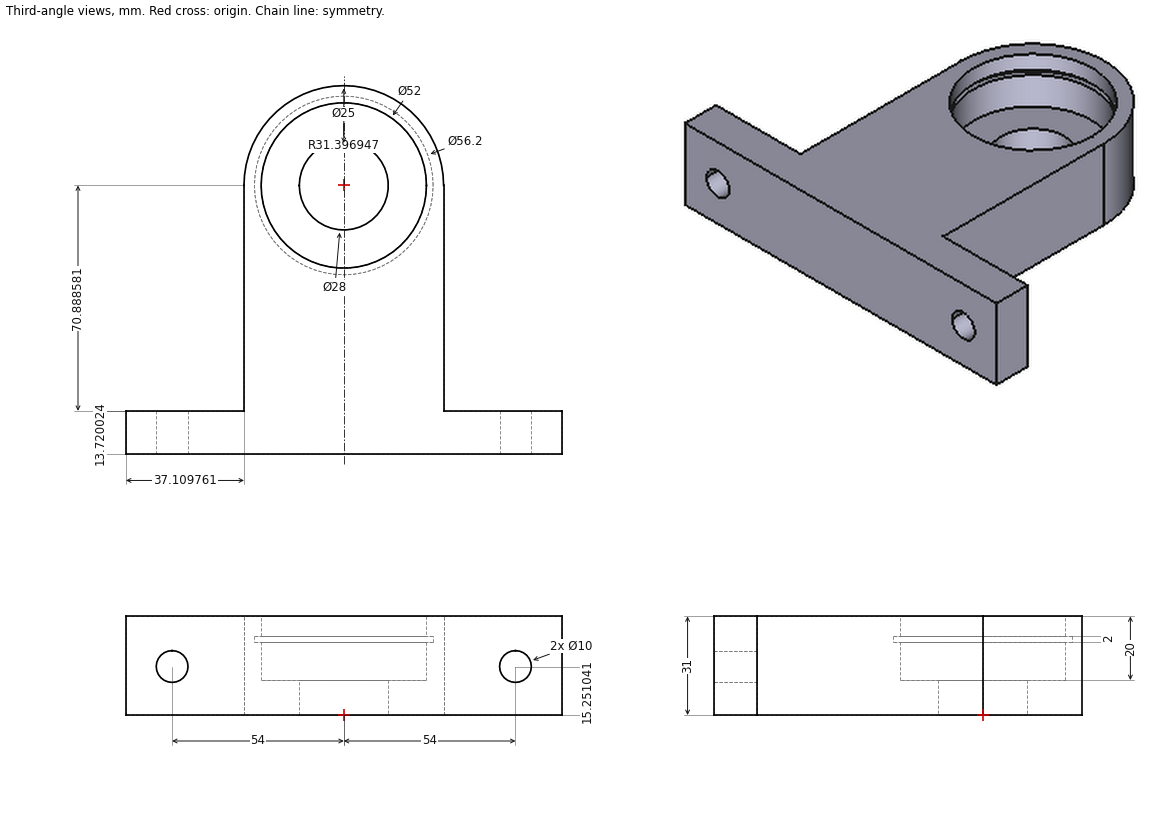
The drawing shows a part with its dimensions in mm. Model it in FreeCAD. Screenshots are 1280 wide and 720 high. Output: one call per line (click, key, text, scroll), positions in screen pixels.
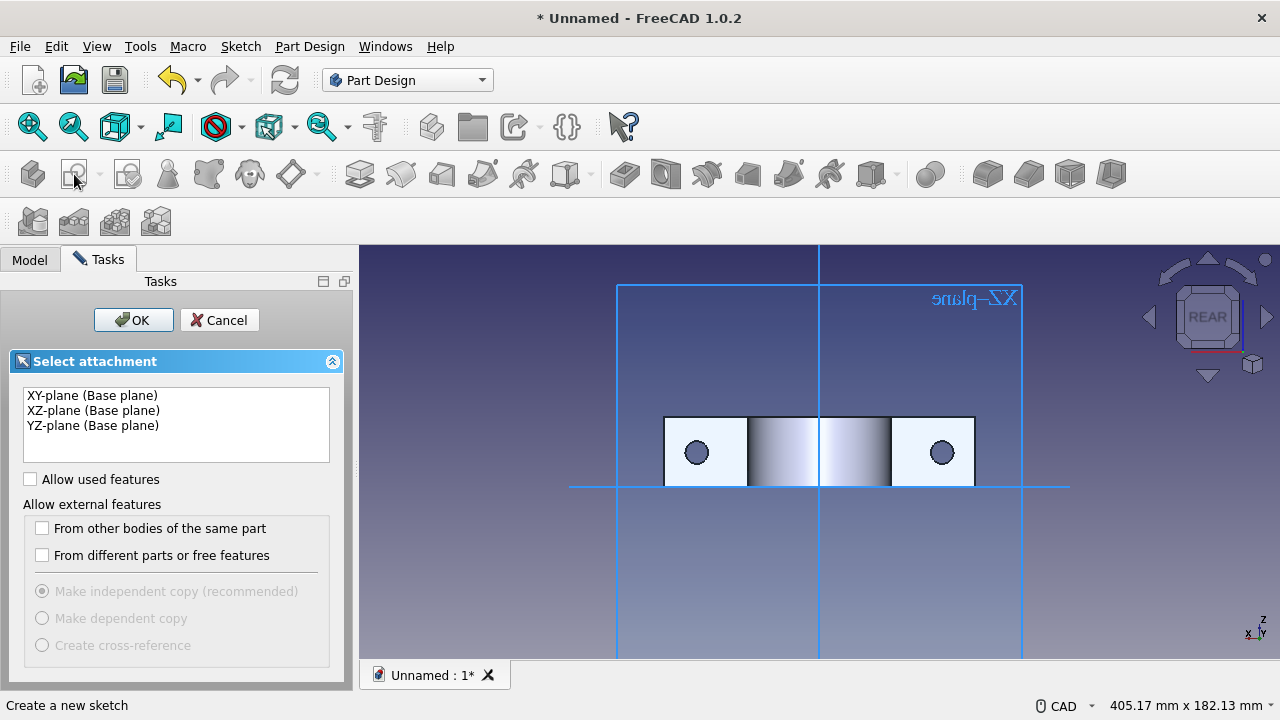
click(84, 396)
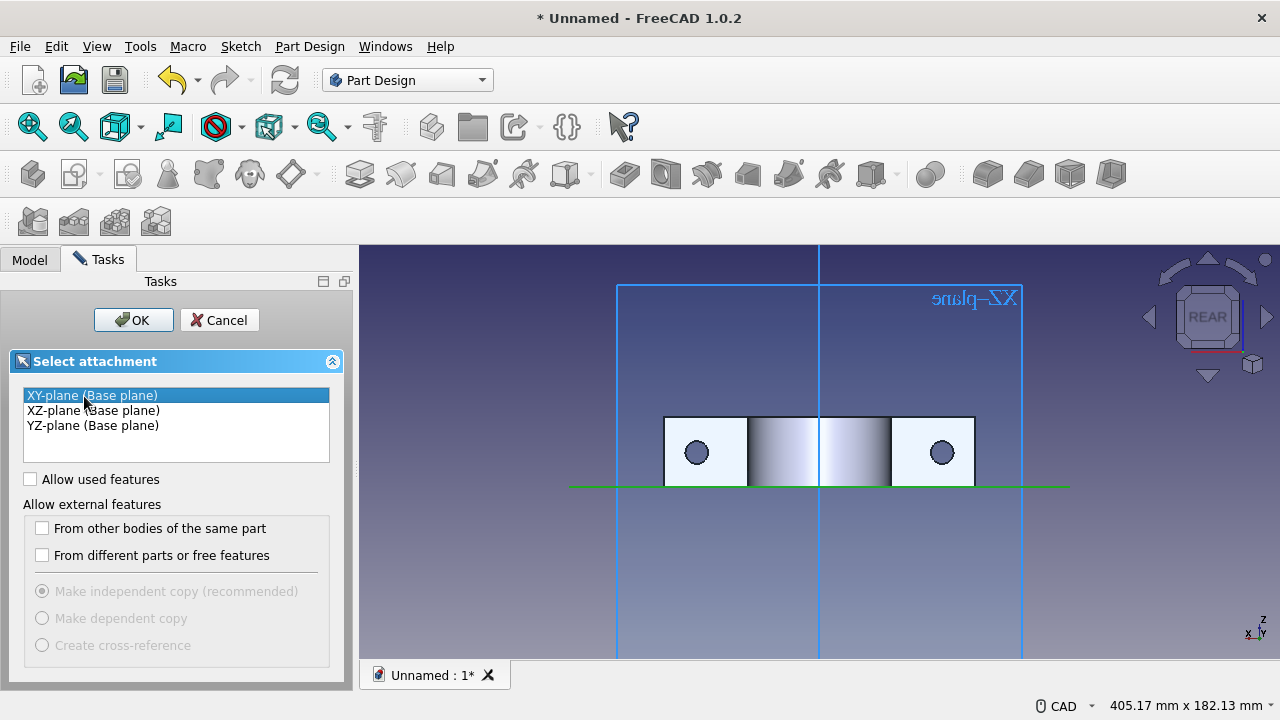
click(134, 320)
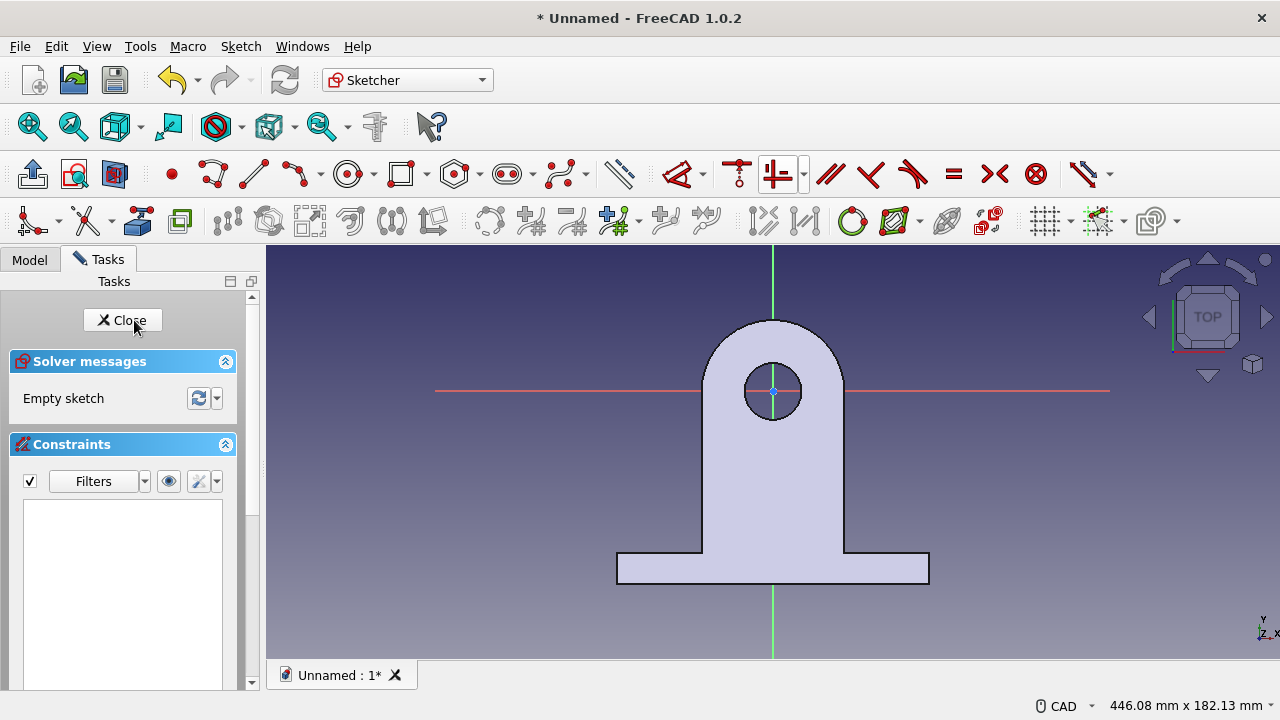
click(115, 174)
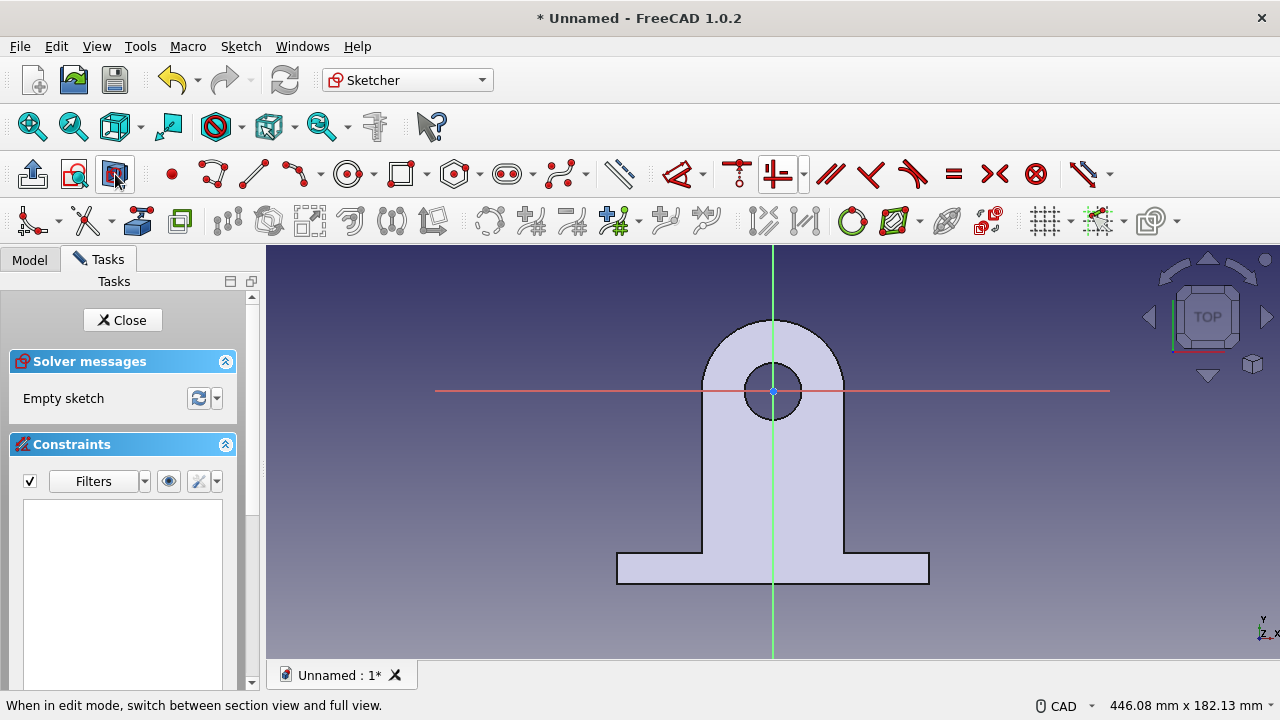
scroll(795, 372, up, 7)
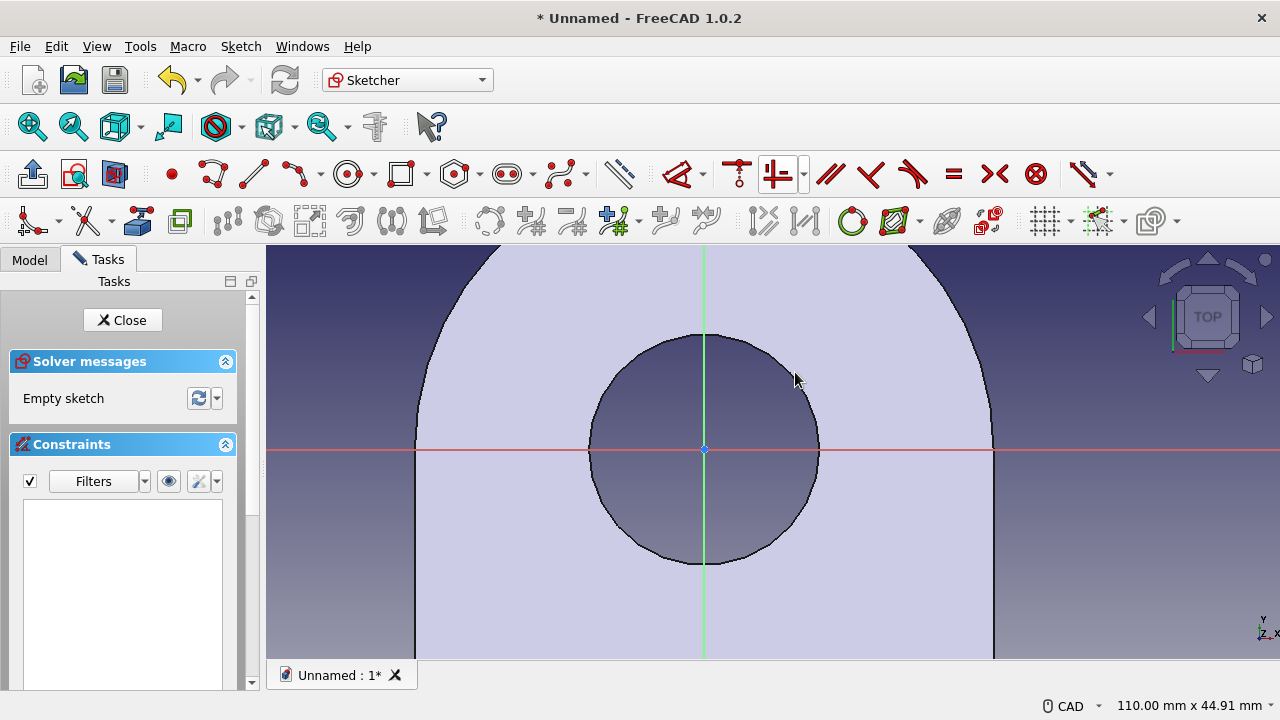
click(348, 174)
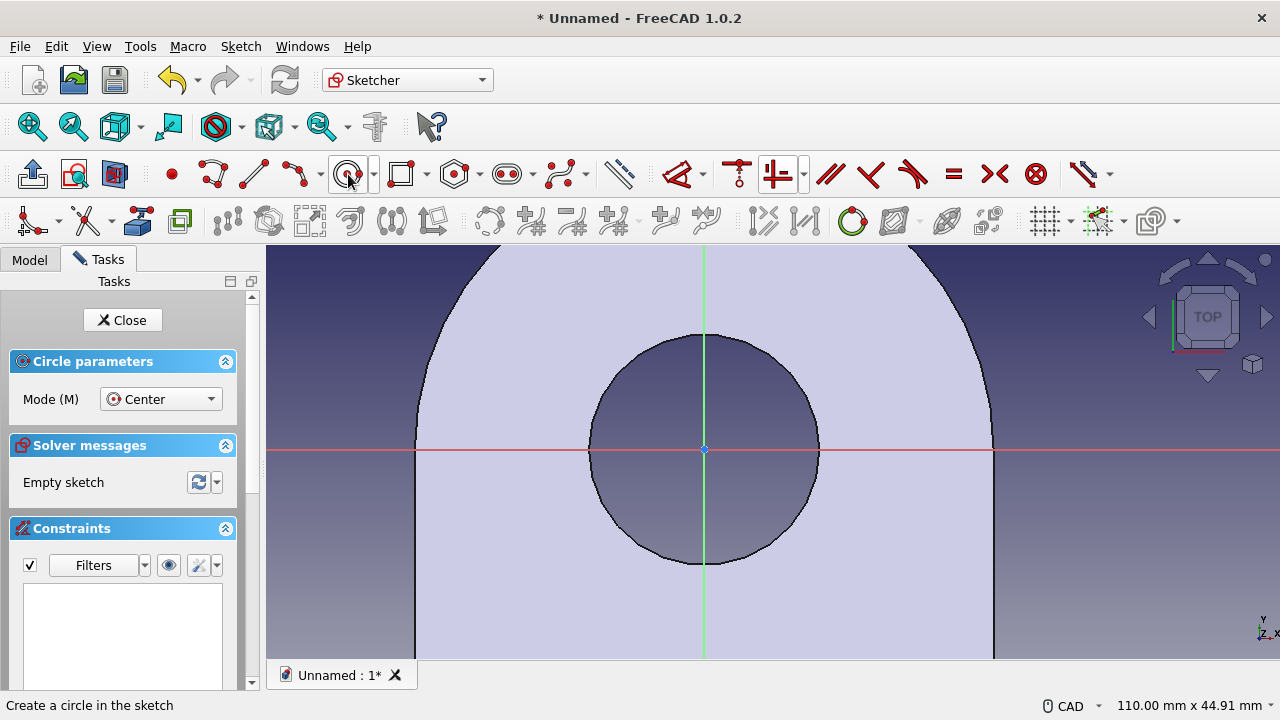
click(704, 450)
click(795, 359)
key(Escape)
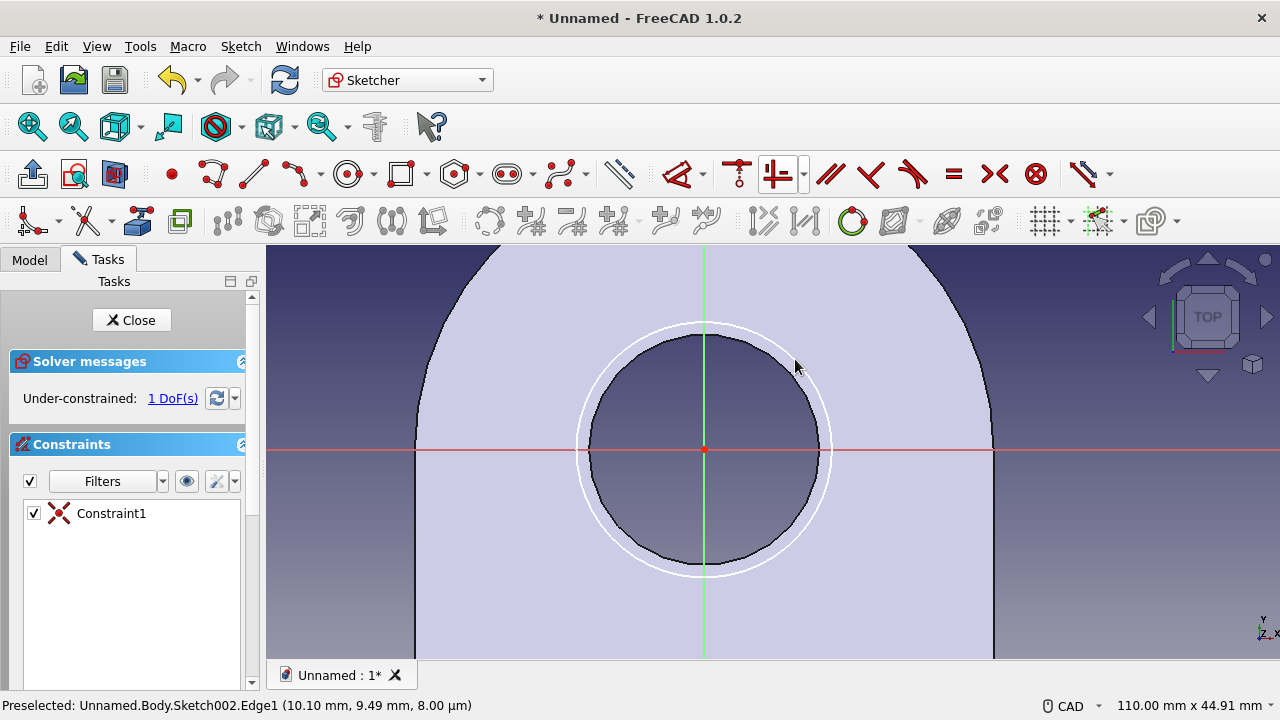
key(d)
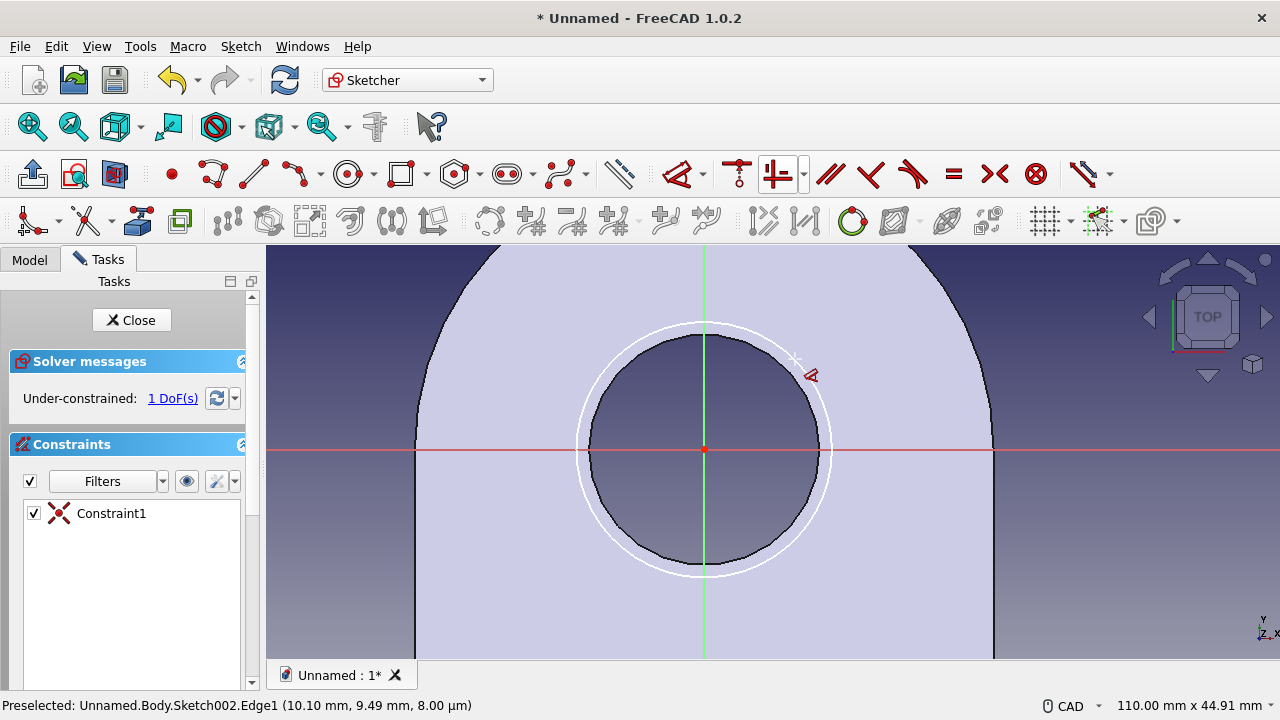
click(794, 359)
click(817, 336)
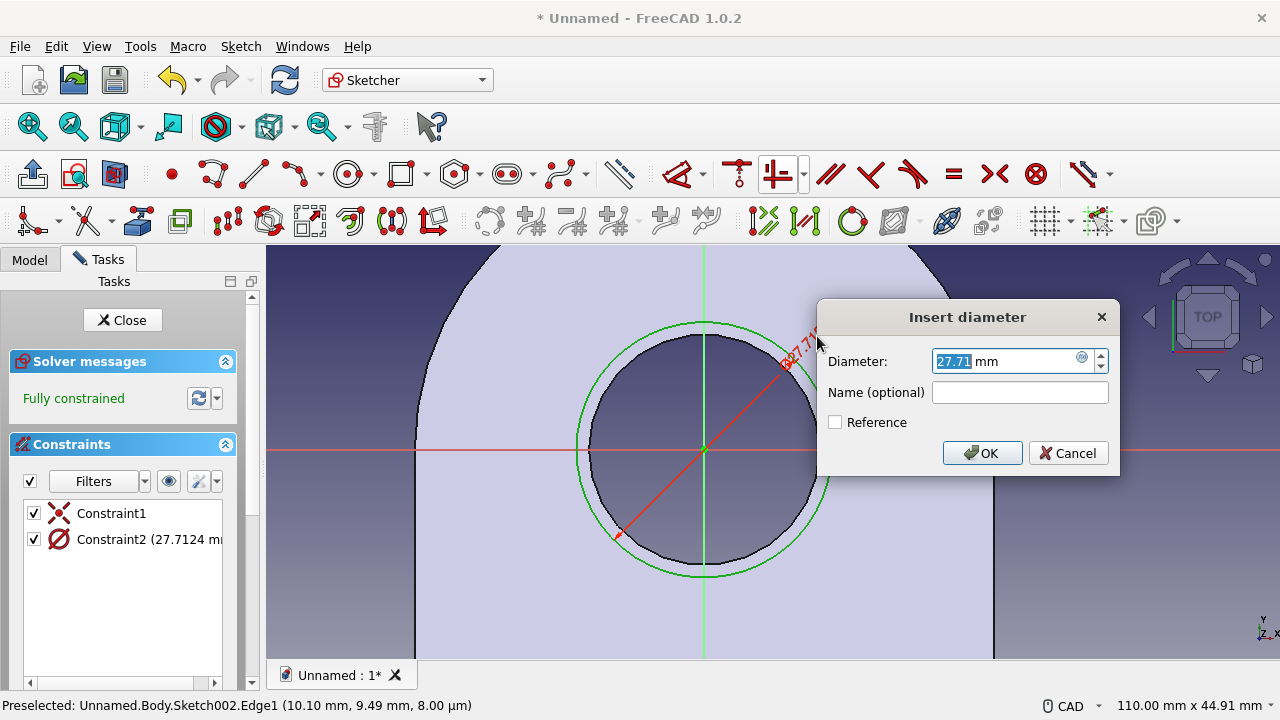
text(28)
key(Return)
key(Escape)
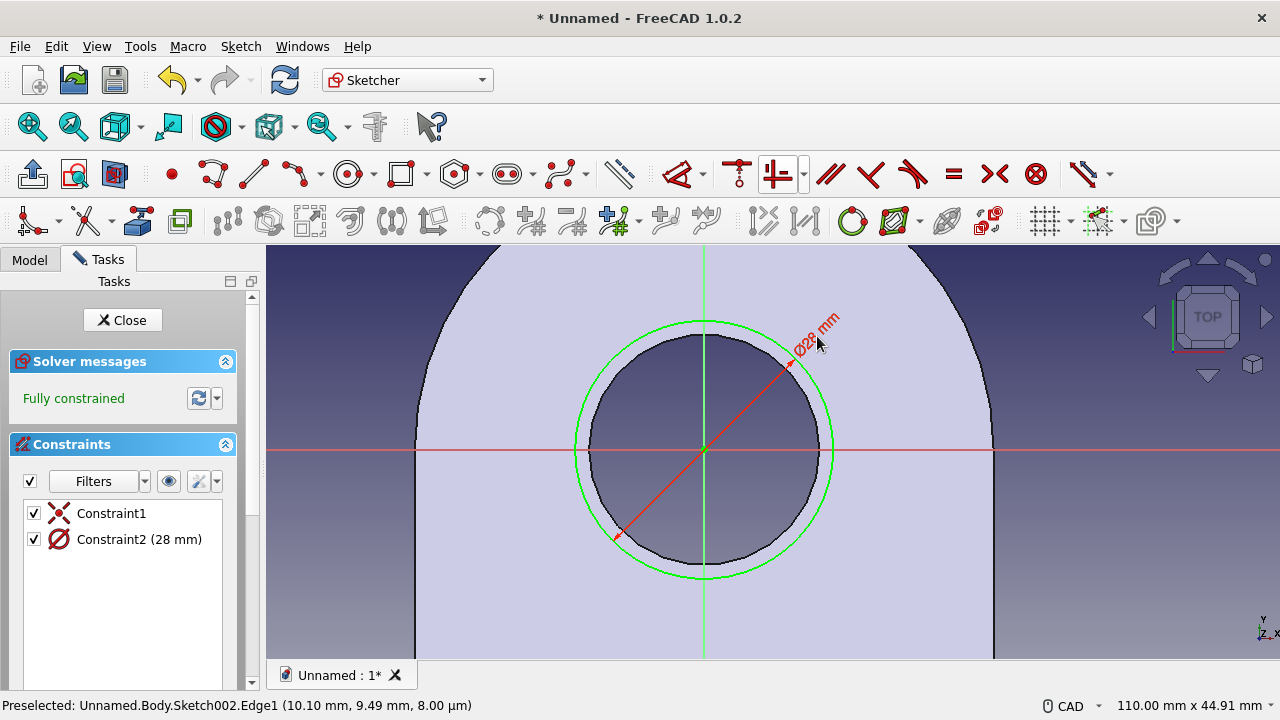
click(123, 320)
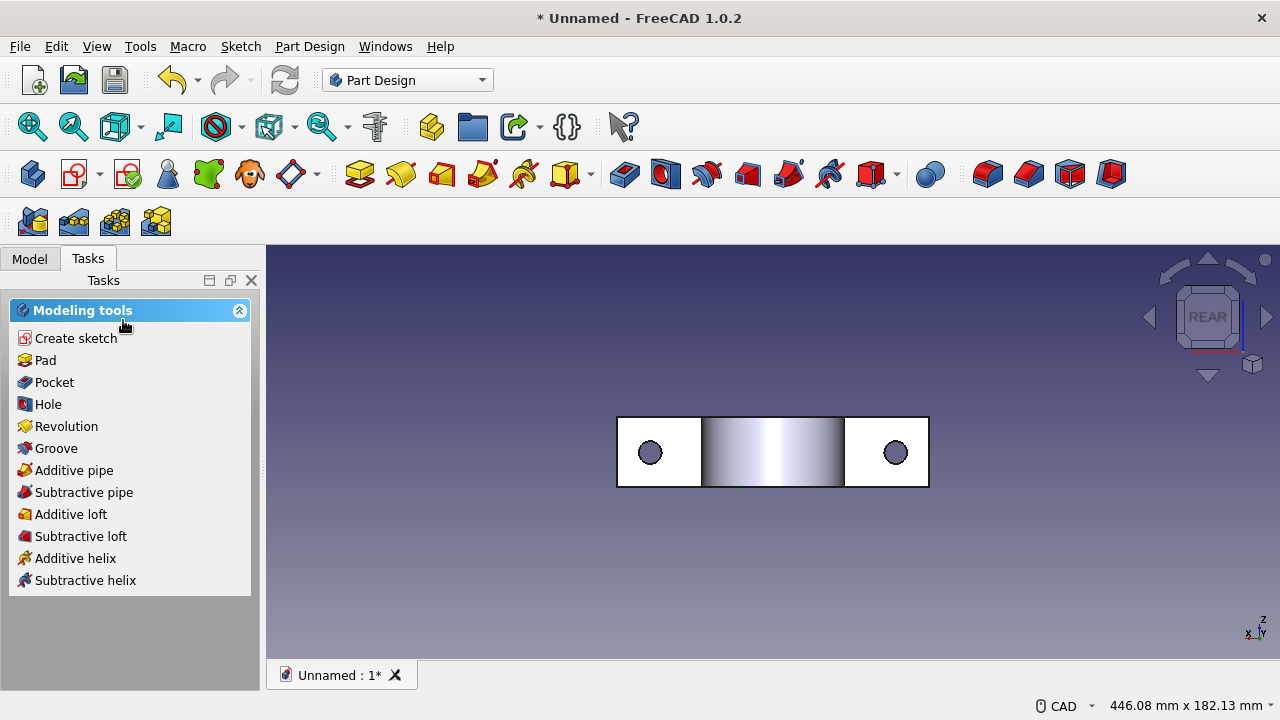
click(625, 174)